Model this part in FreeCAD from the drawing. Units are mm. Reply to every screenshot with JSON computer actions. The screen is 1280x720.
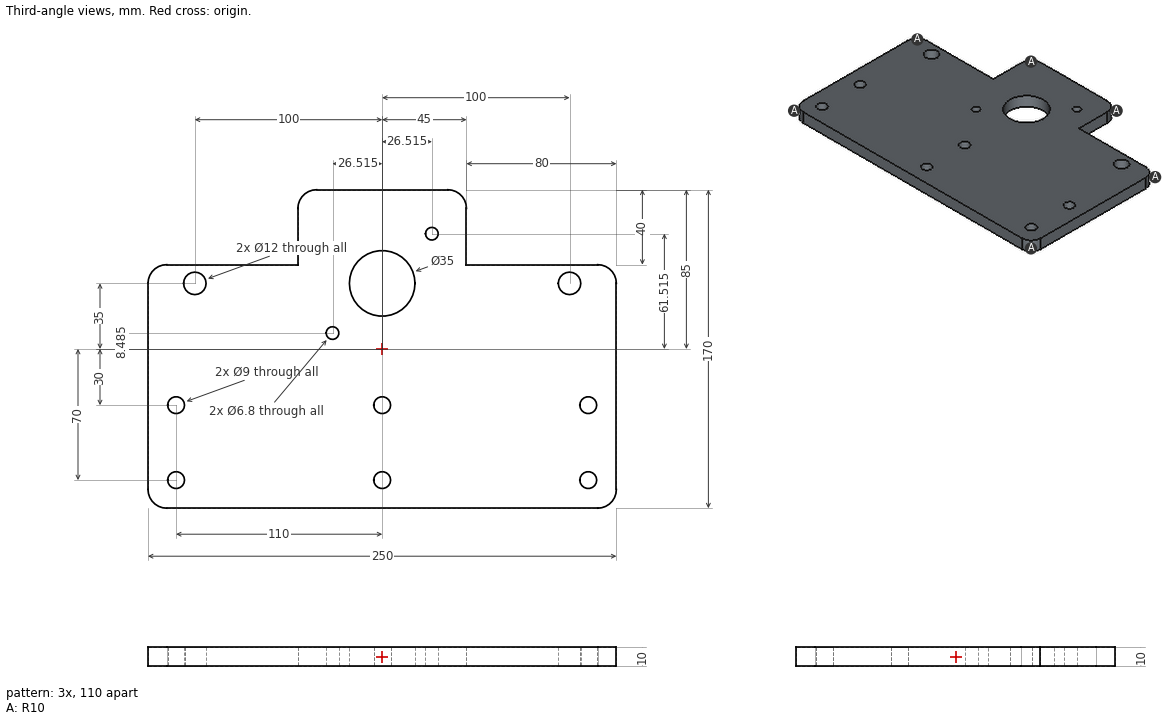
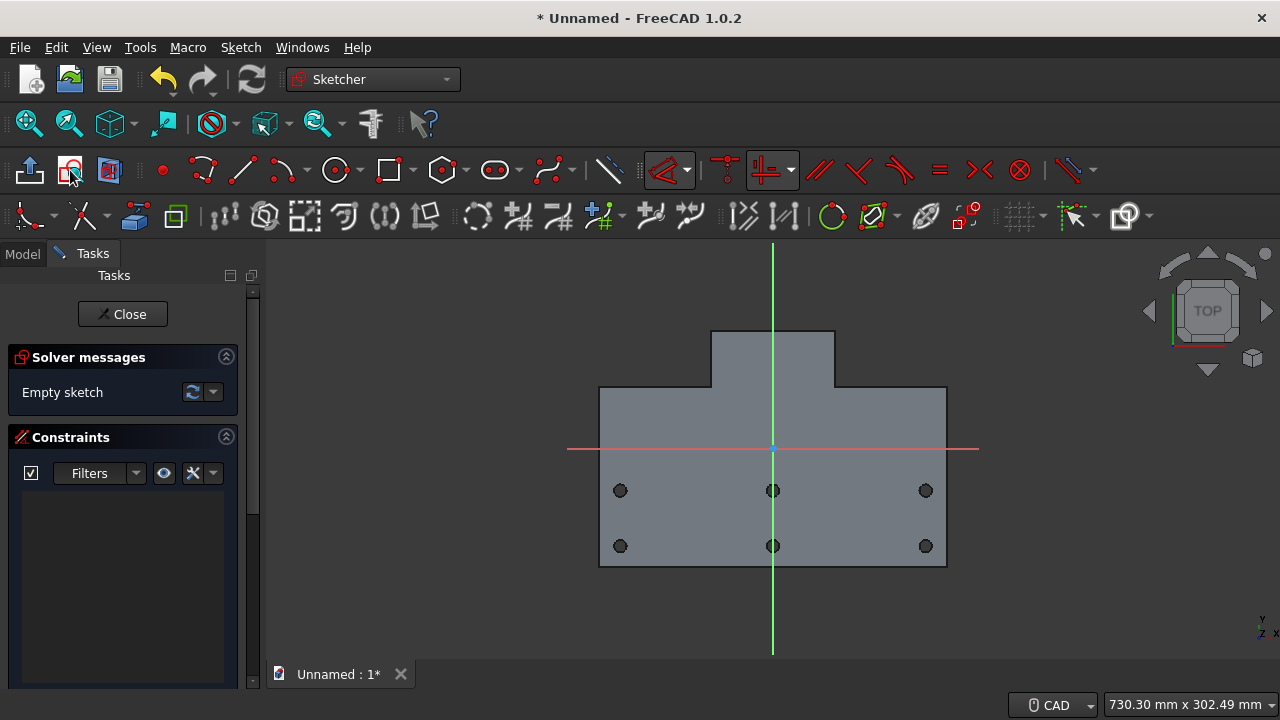
{"action": "scroll", "coordinate": [856, 386], "scroll_direction": "up", "scroll_amount": 3}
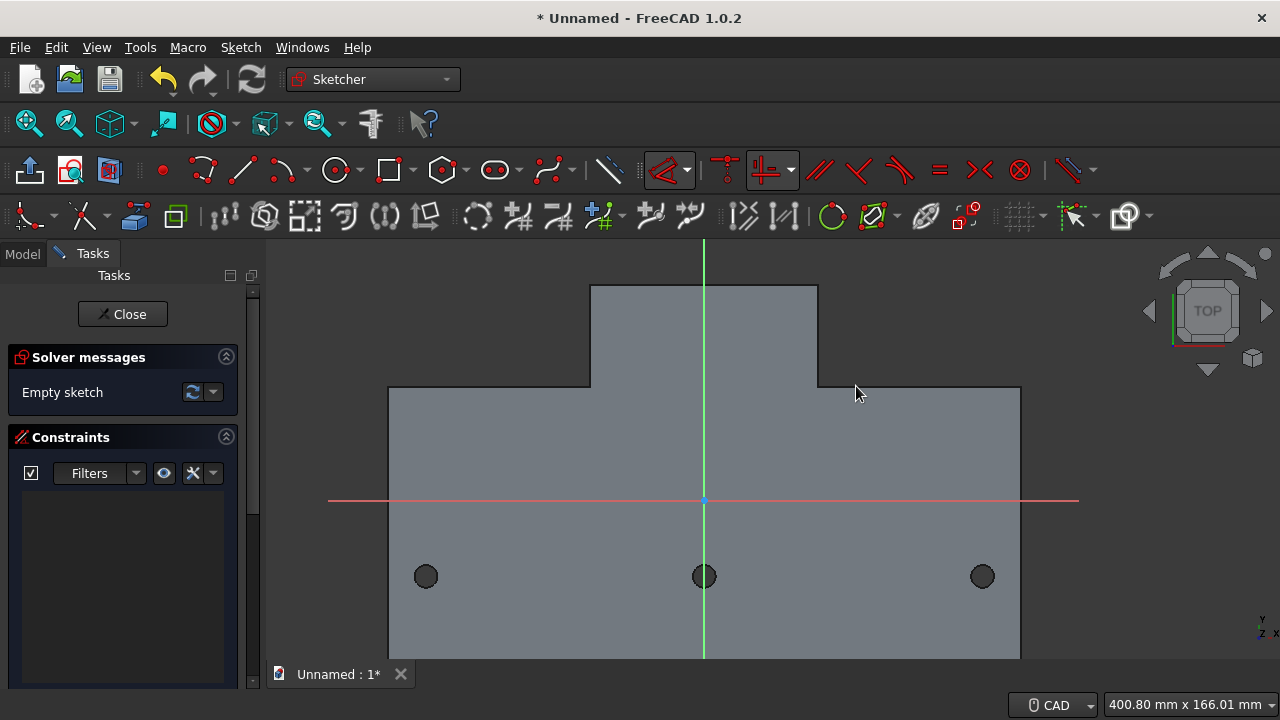
{"action": "left_click", "coordinate": [336, 170]}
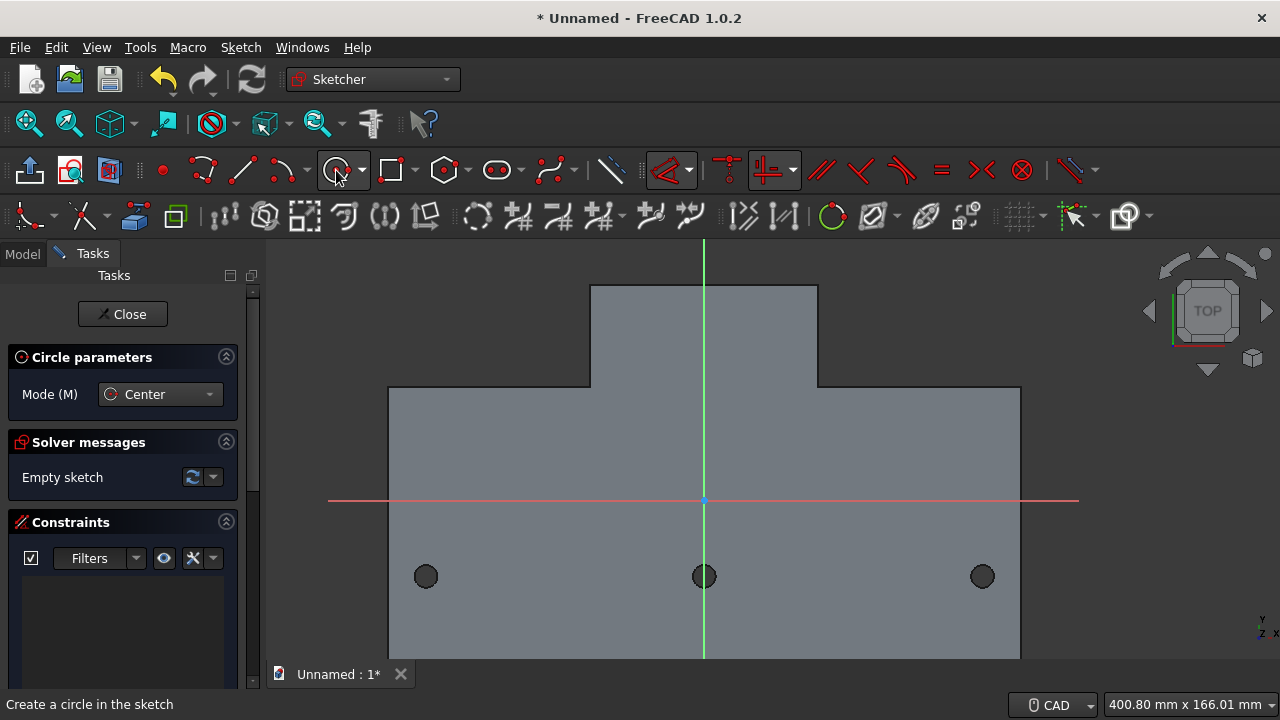
{"action": "scroll", "coordinate": [451, 412], "scroll_direction": "up", "scroll_amount": 3}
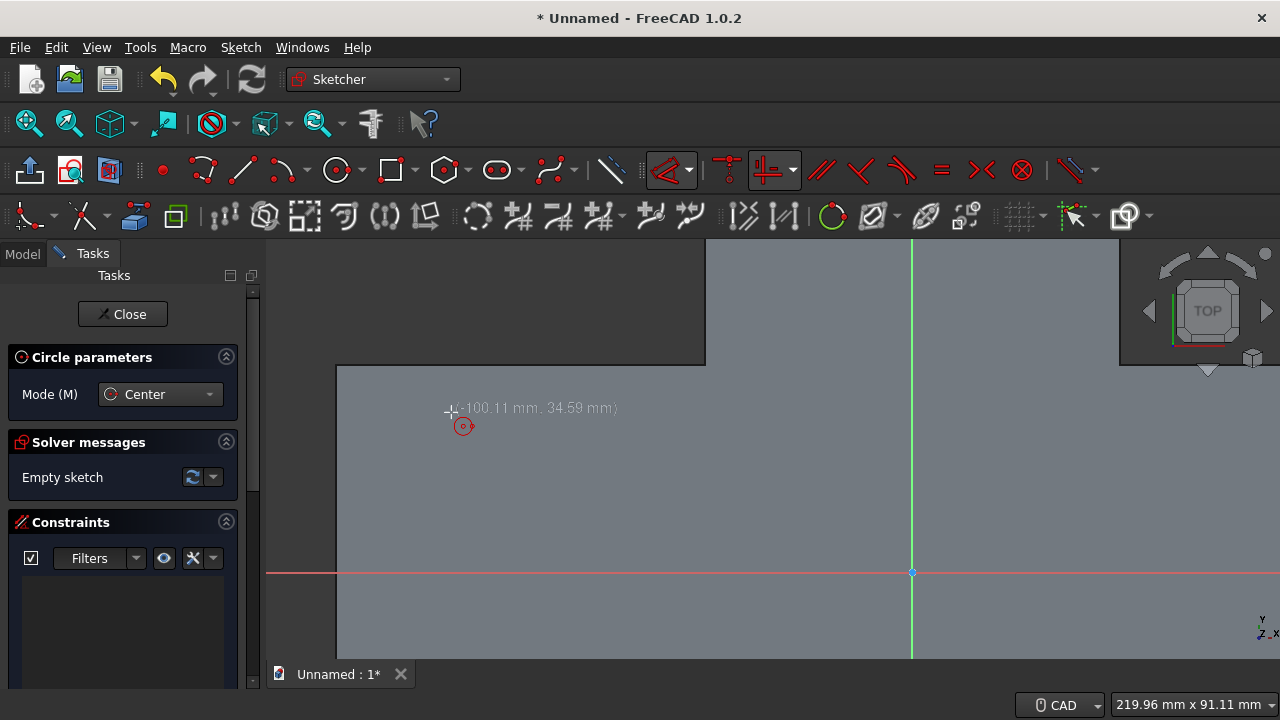
{"action": "left_click", "coordinate": [451, 412]}
{"action": "mouse_move", "coordinate": [471, 392]}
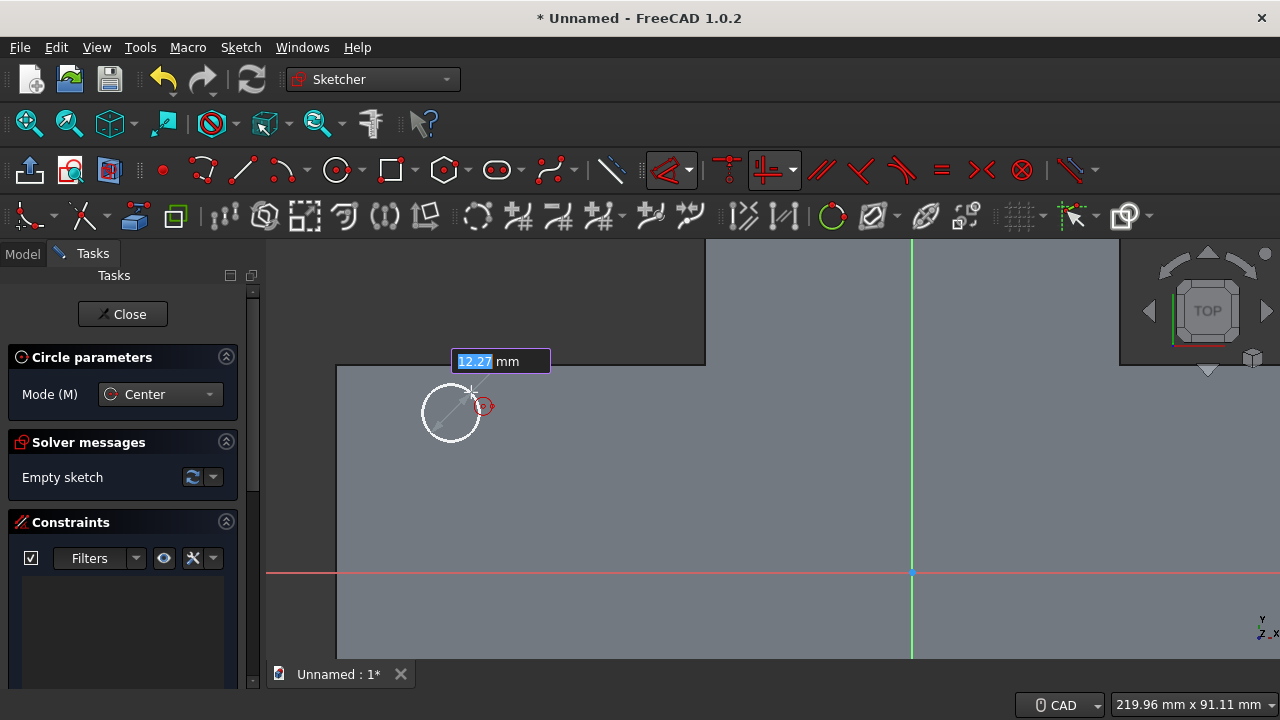
{"action": "type", "text": "12"}
{"action": "key", "text": "Return"}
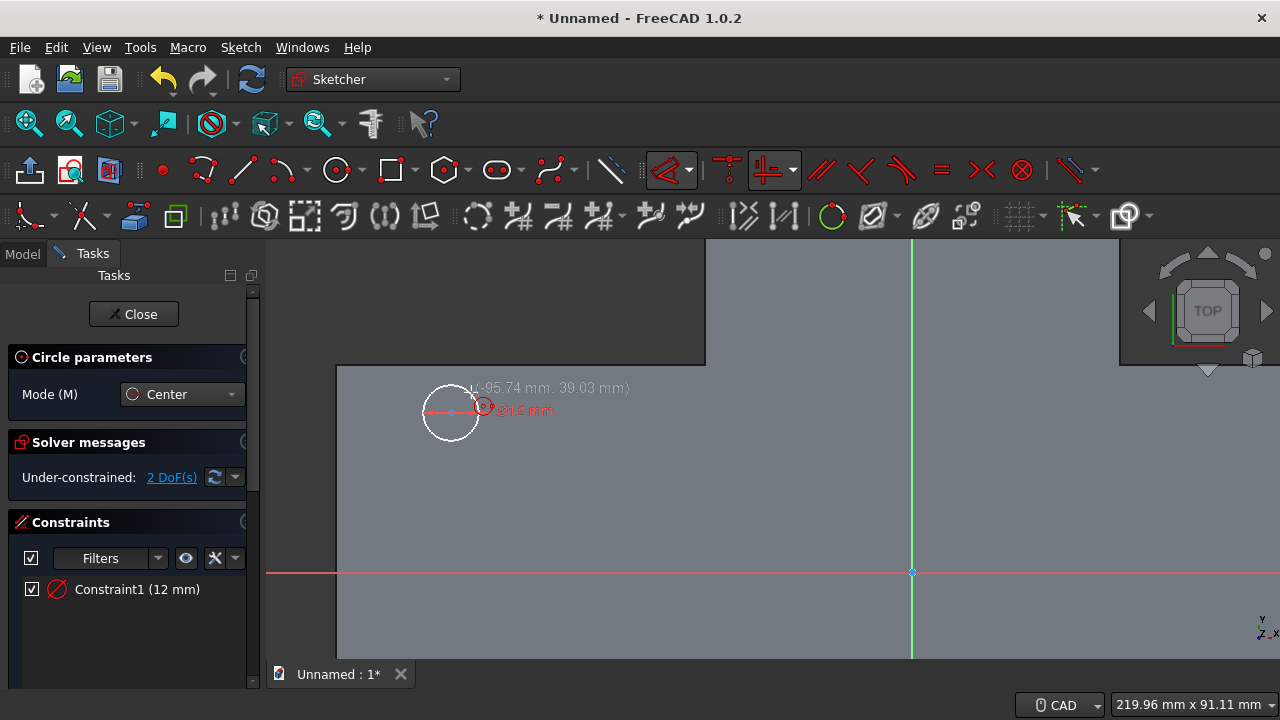
{"action": "scroll", "coordinate": [452, 413], "scroll_direction": "down", "scroll_amount": 3}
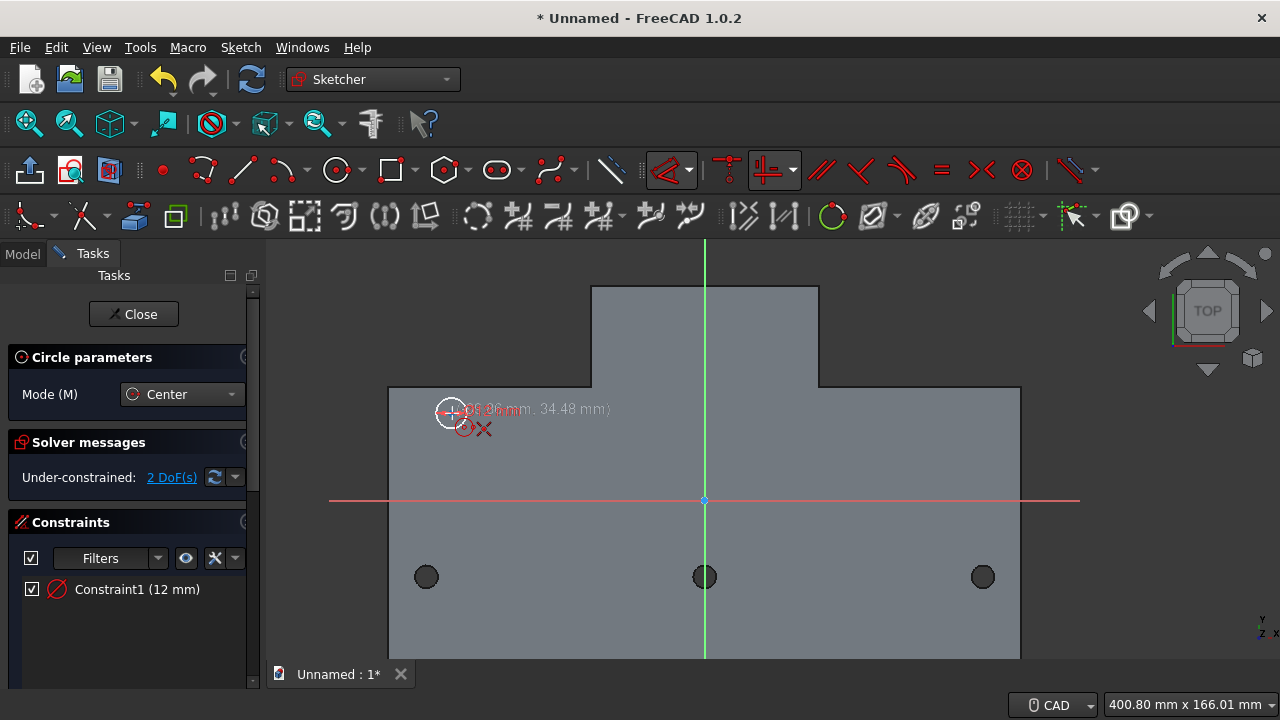
{"action": "scroll", "coordinate": [958, 412], "scroll_direction": "up", "scroll_amount": 3}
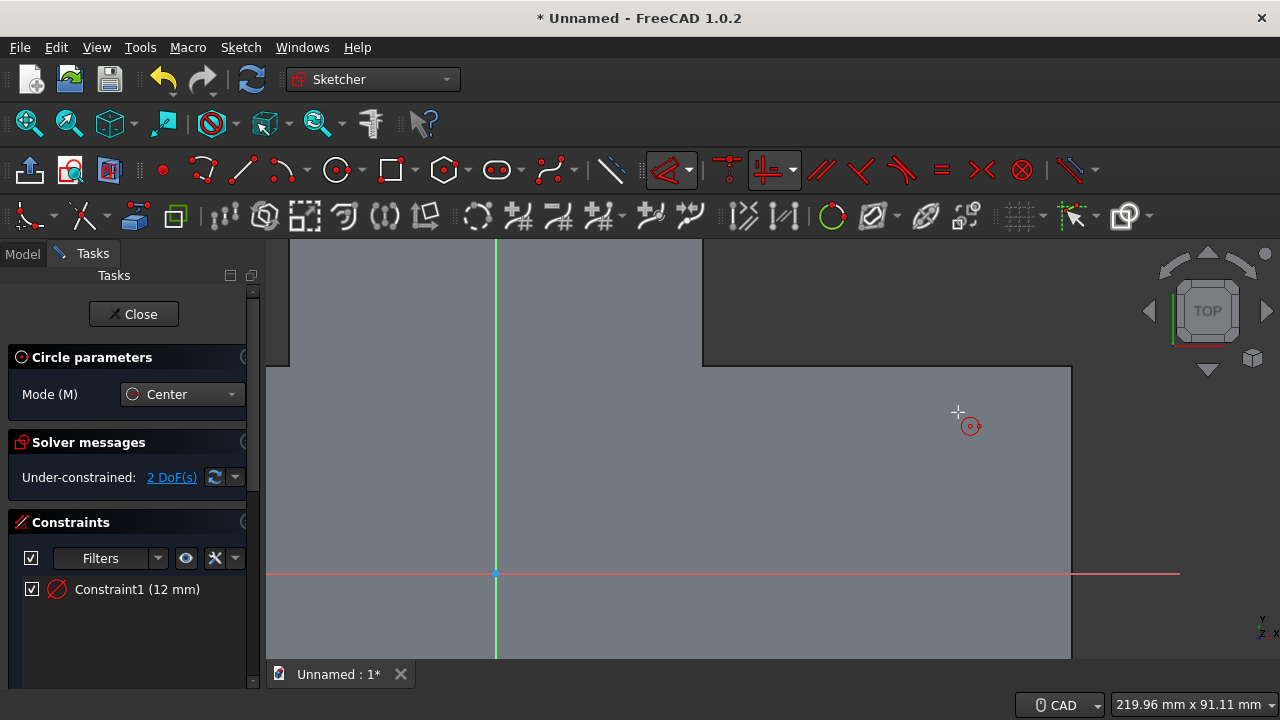
{"action": "left_click", "coordinate": [957, 412]}
{"action": "mouse_move", "coordinate": [977, 393]}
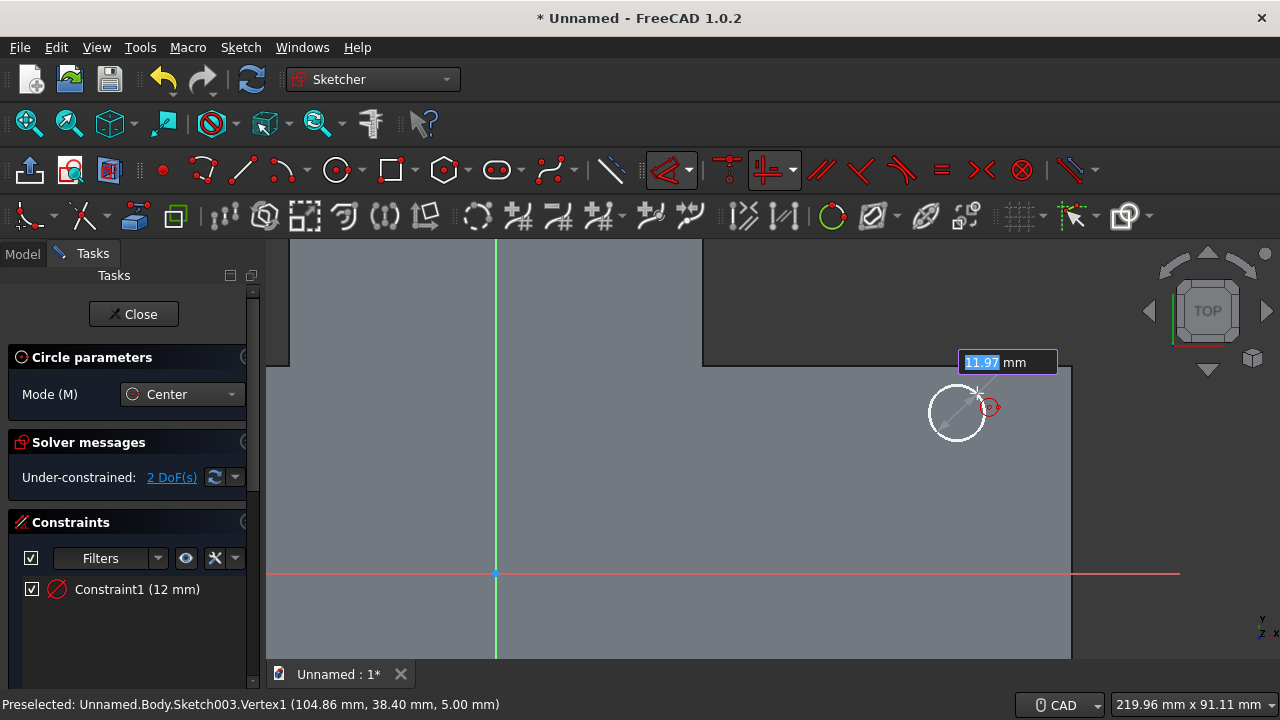
{"action": "type", "text": "12"}
{"action": "key", "text": "Return"}
{"action": "key", "text": "Escape"}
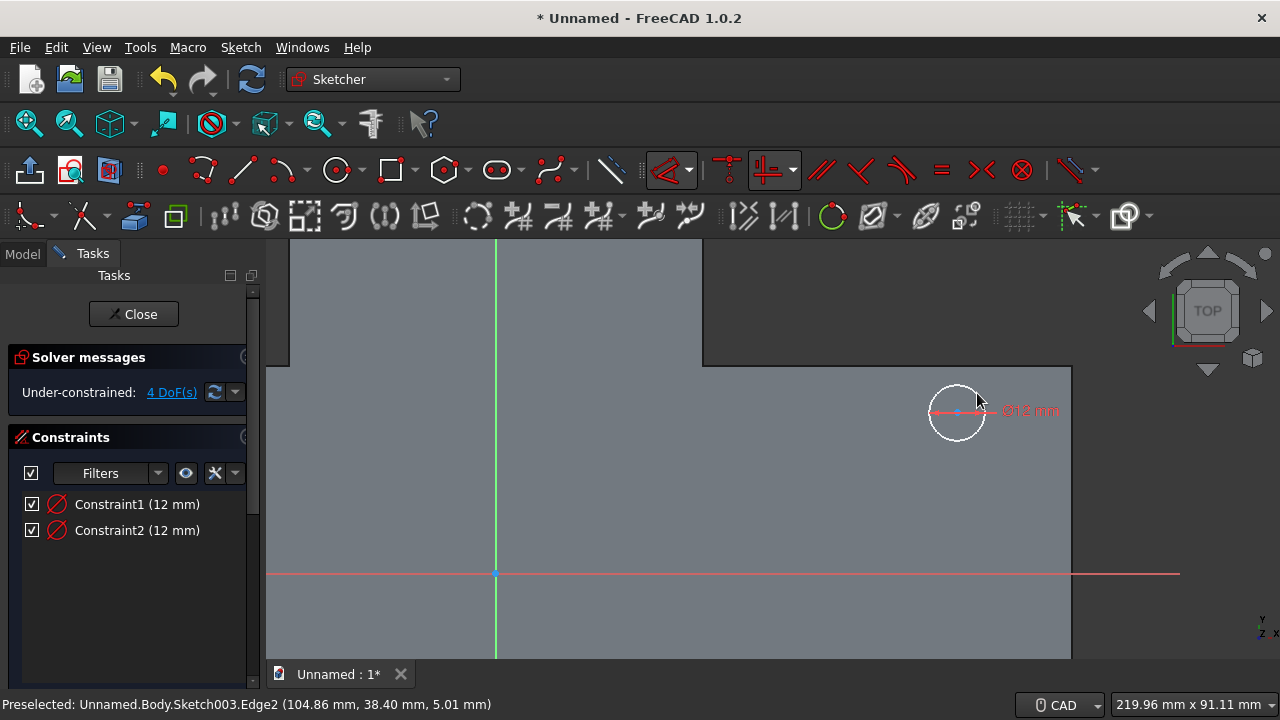
{"action": "scroll", "coordinate": [958, 412], "scroll_direction": "down", "scroll_amount": 3}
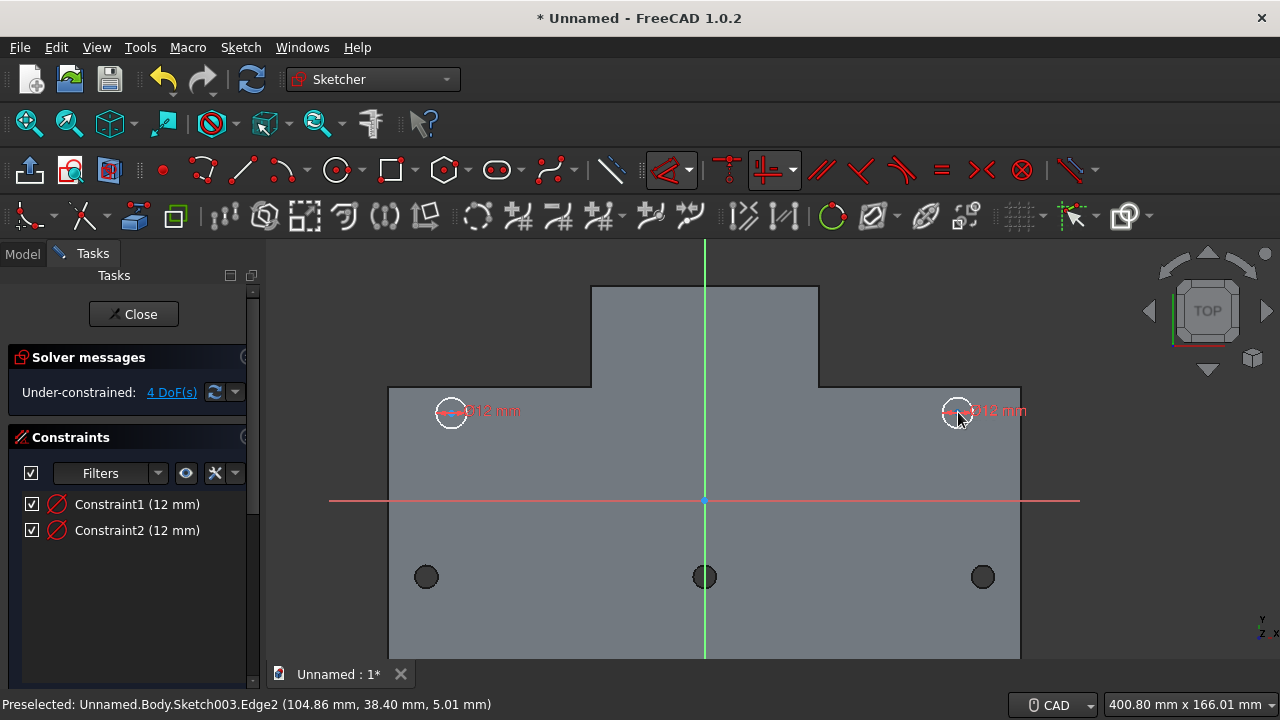
{"action": "left_click", "coordinate": [452, 413]}